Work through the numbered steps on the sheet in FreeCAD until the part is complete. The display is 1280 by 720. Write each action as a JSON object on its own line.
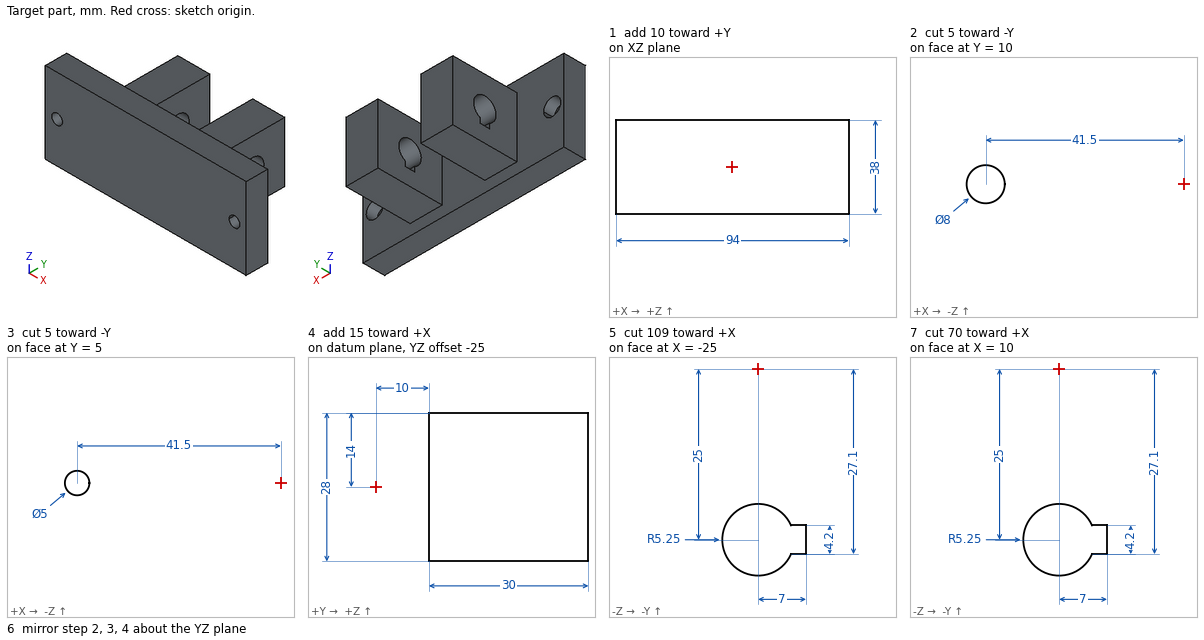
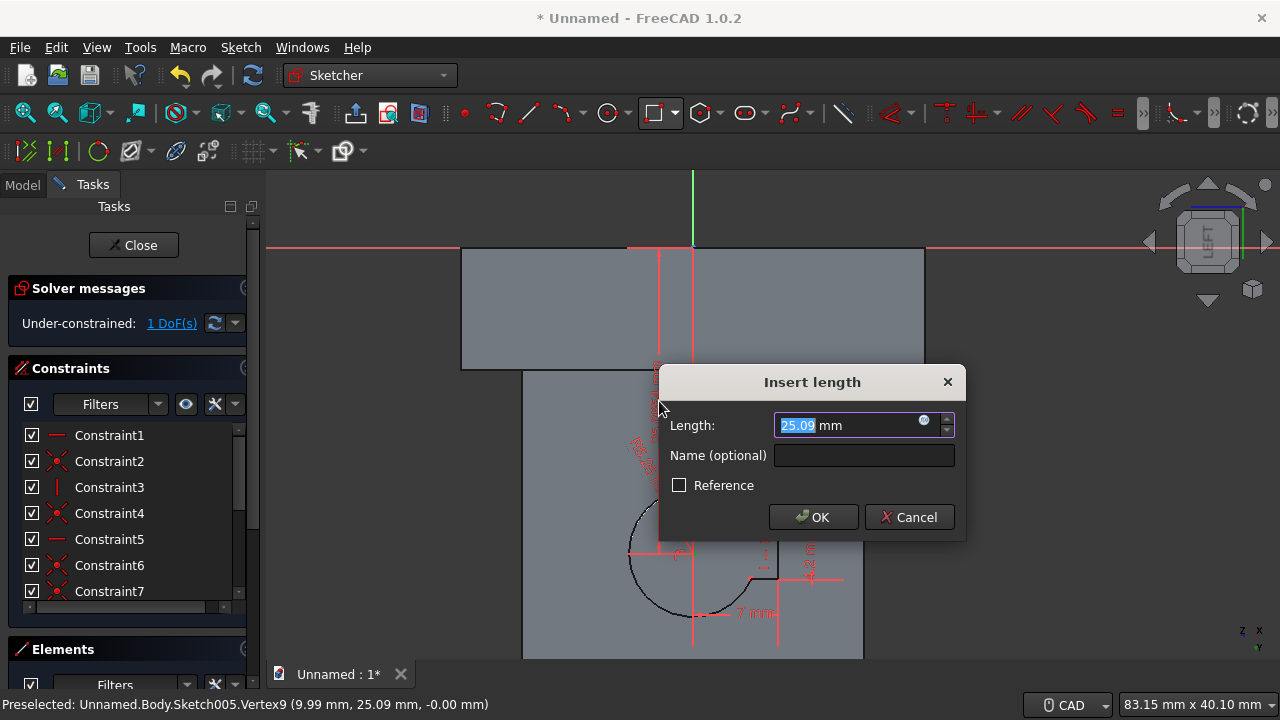
{"action": "type", "text": "25"}
{"action": "key", "text": "Return"}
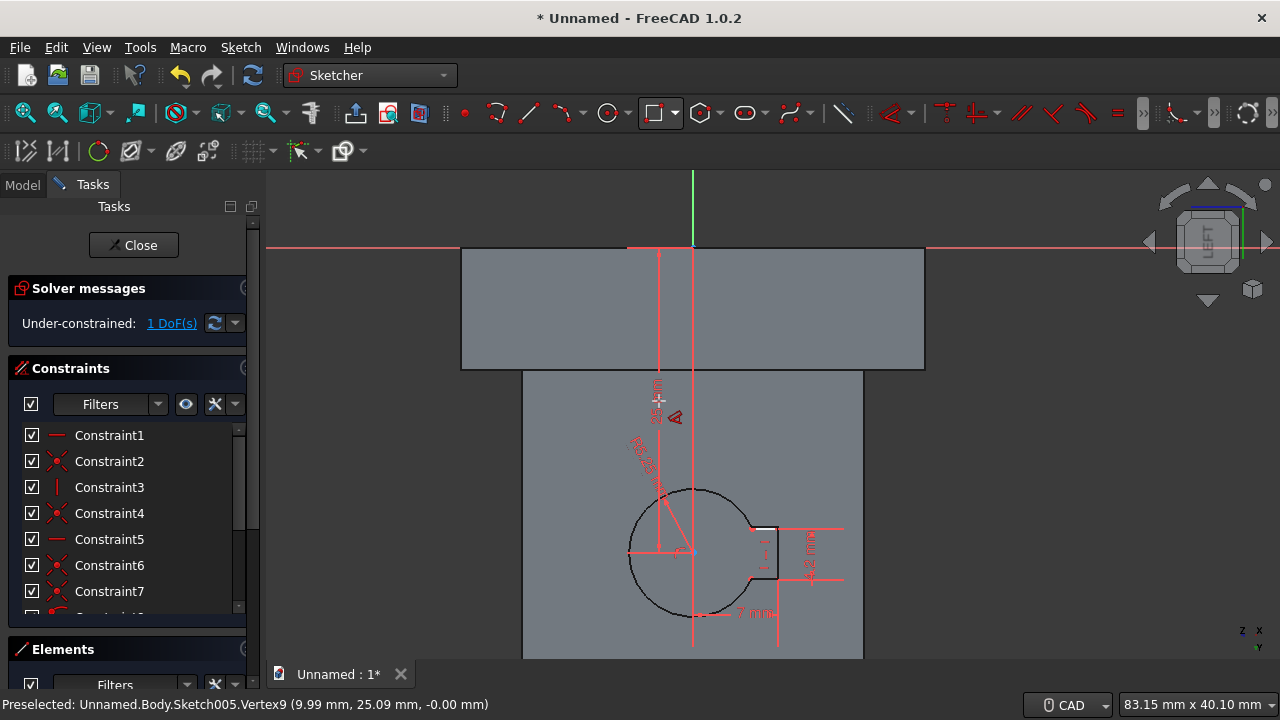
{"action": "left_click", "coordinate": [751, 580]}
{"action": "left_click", "coordinate": [785, 414]}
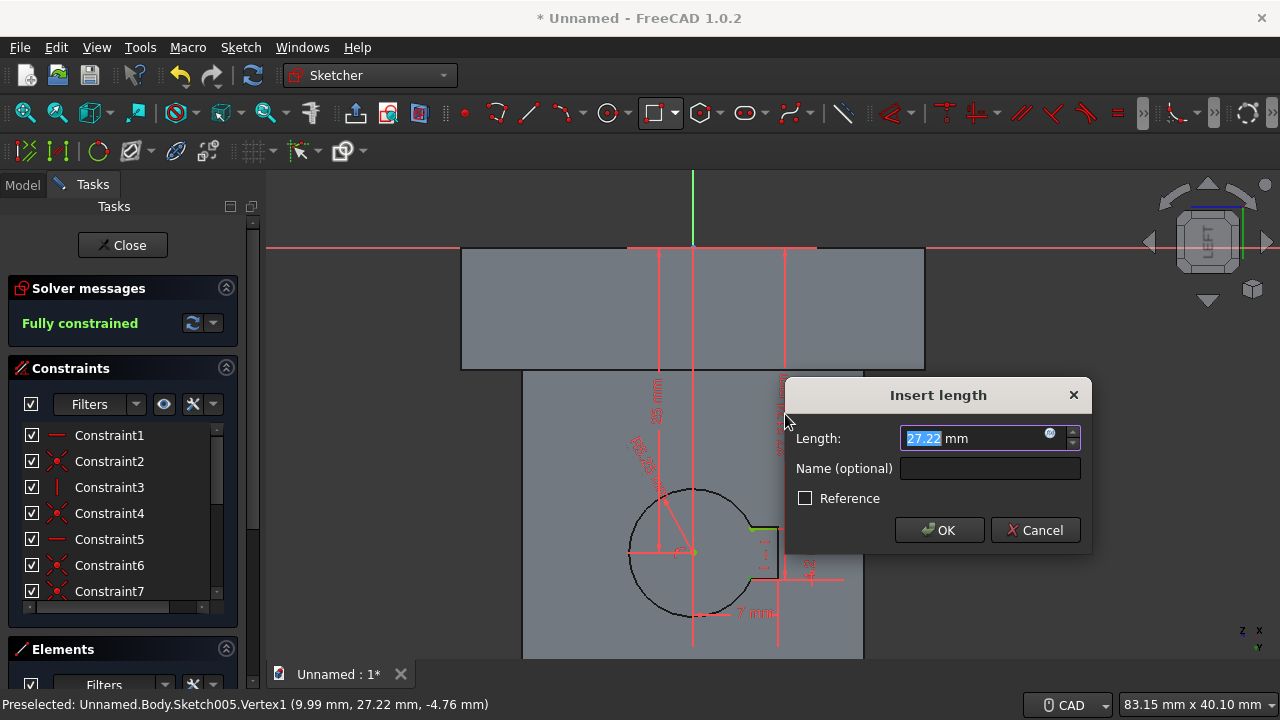
{"action": "type", "text": "27.1"}
{"action": "key", "text": "Return"}
{"action": "key", "text": "Escape"}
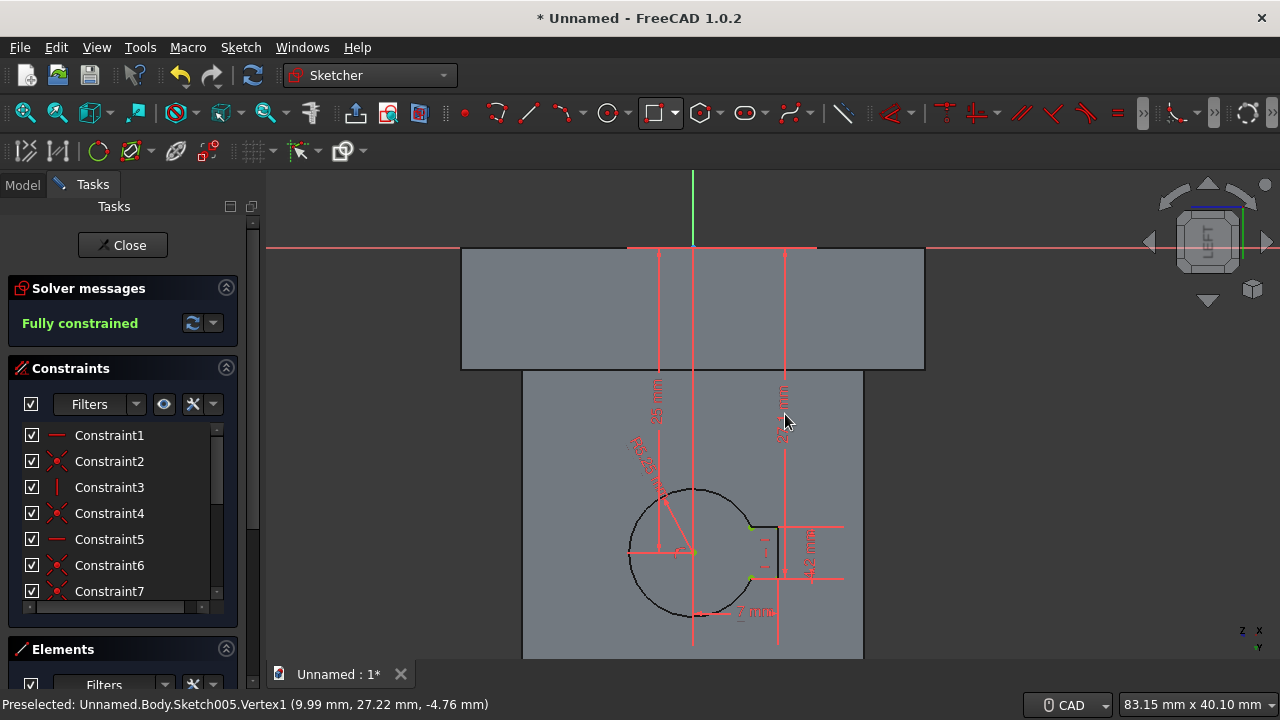
{"action": "left_click", "coordinate": [123, 245]}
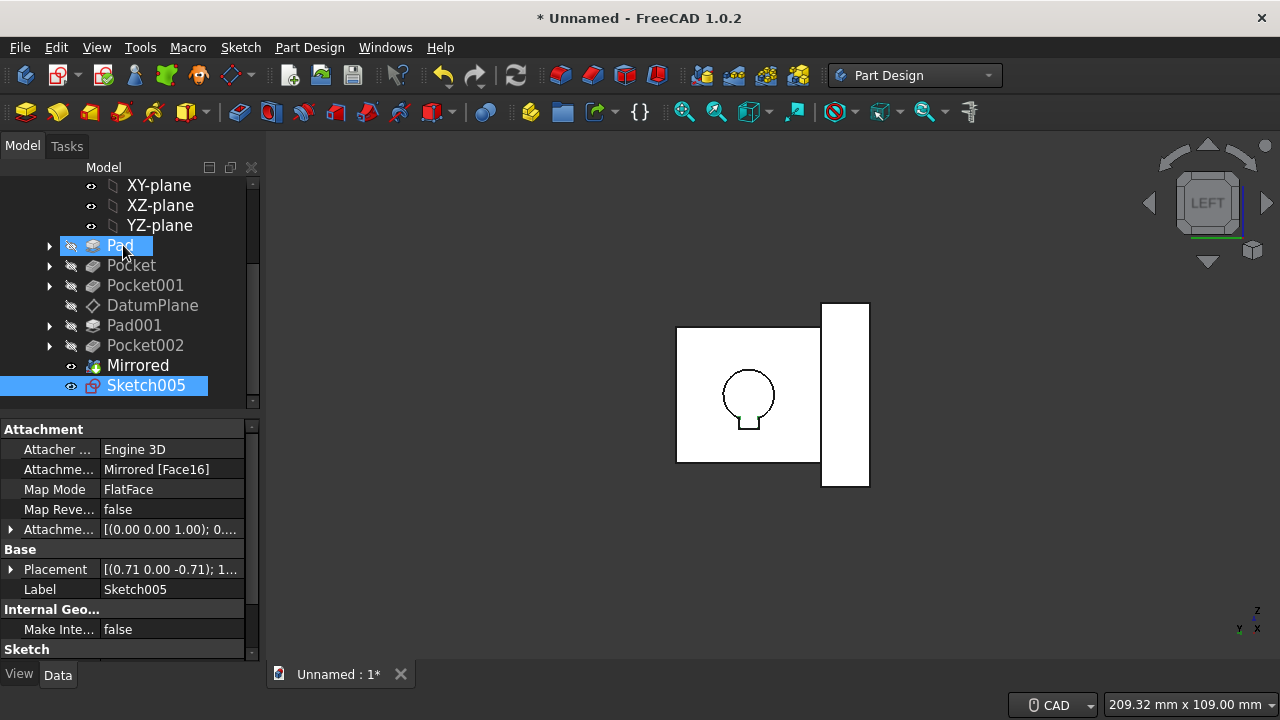
{"action": "left_click", "coordinate": [240, 112]}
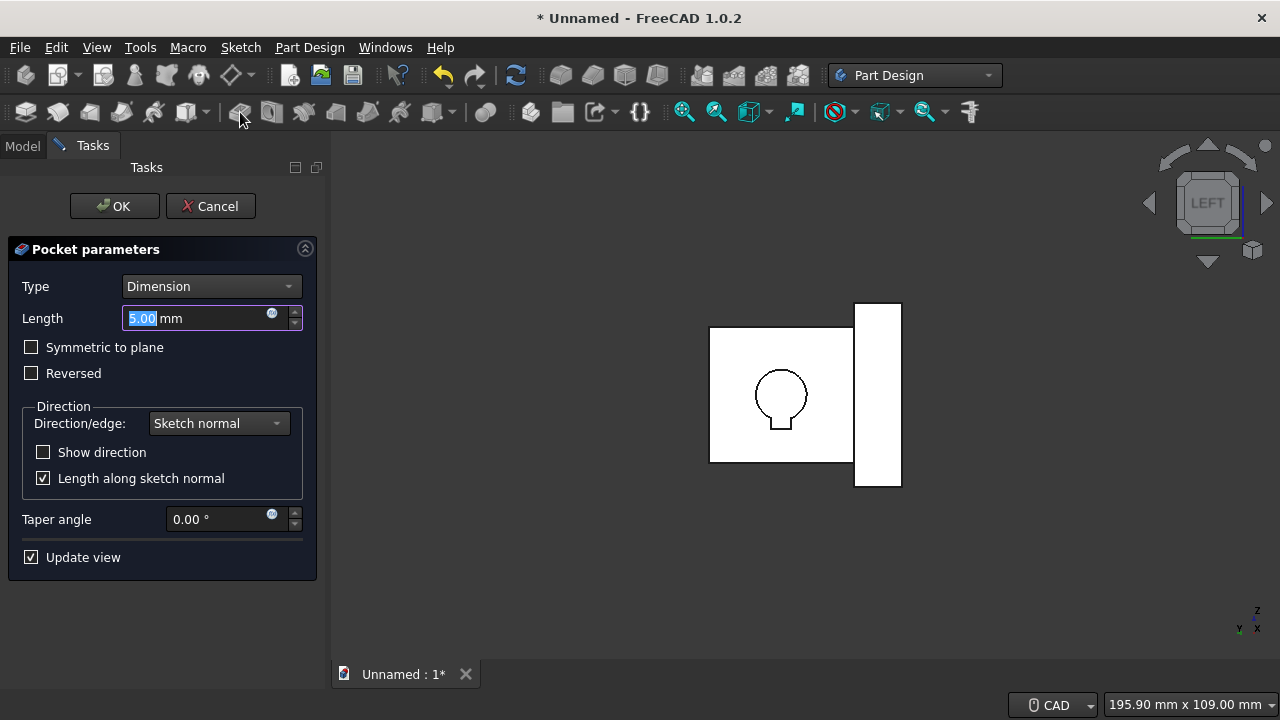
{"action": "type", "text": "70"}
{"action": "key", "text": "Tab"}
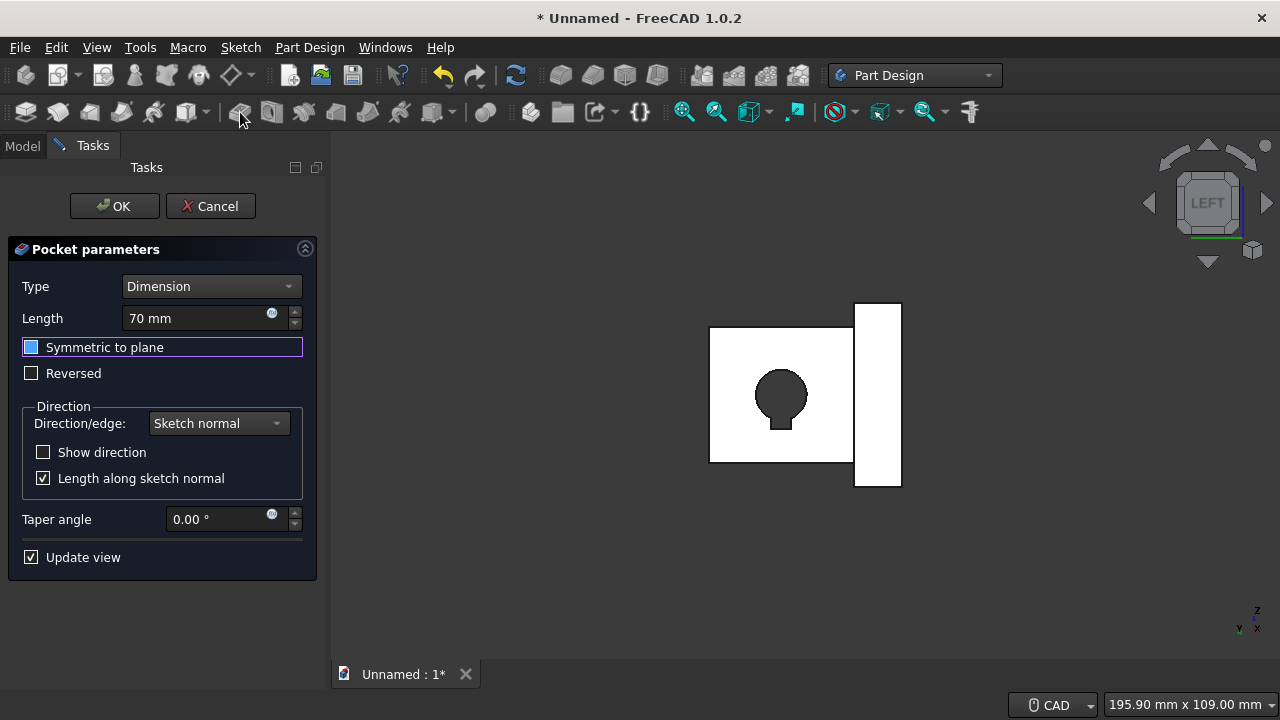
{"action": "left_click", "coordinate": [115, 206]}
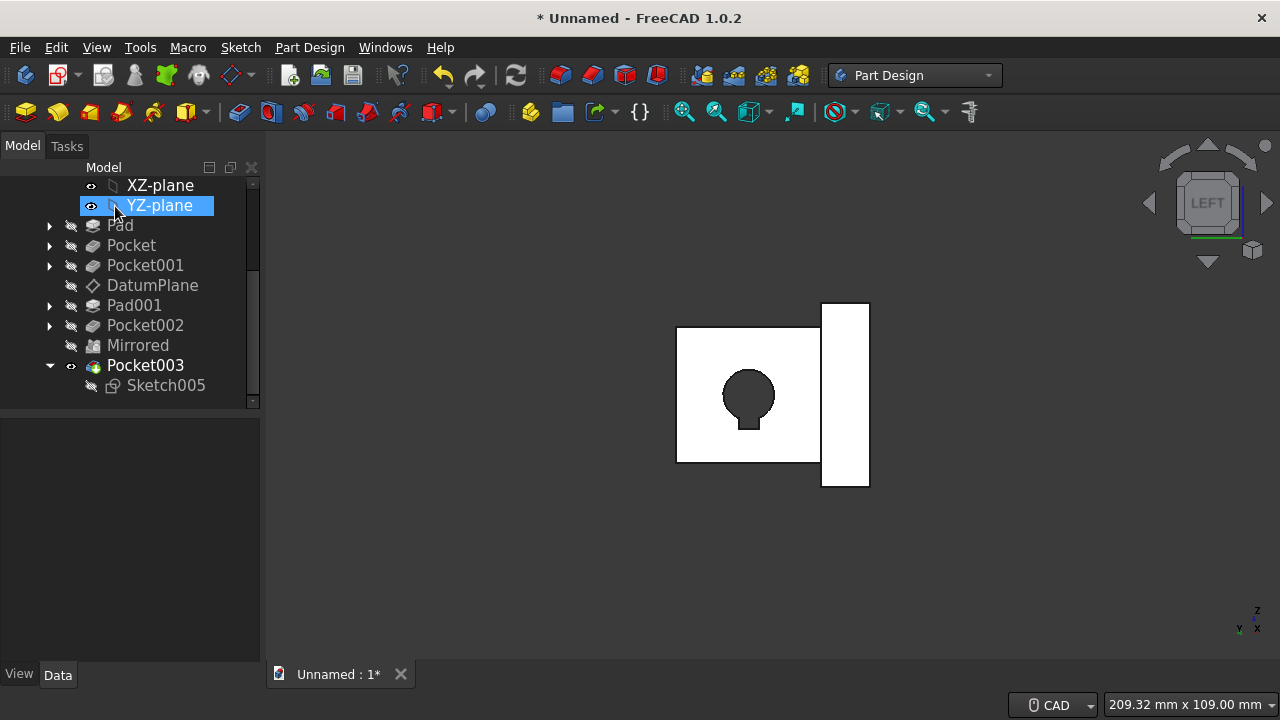
{"action": "key", "text": "0"}